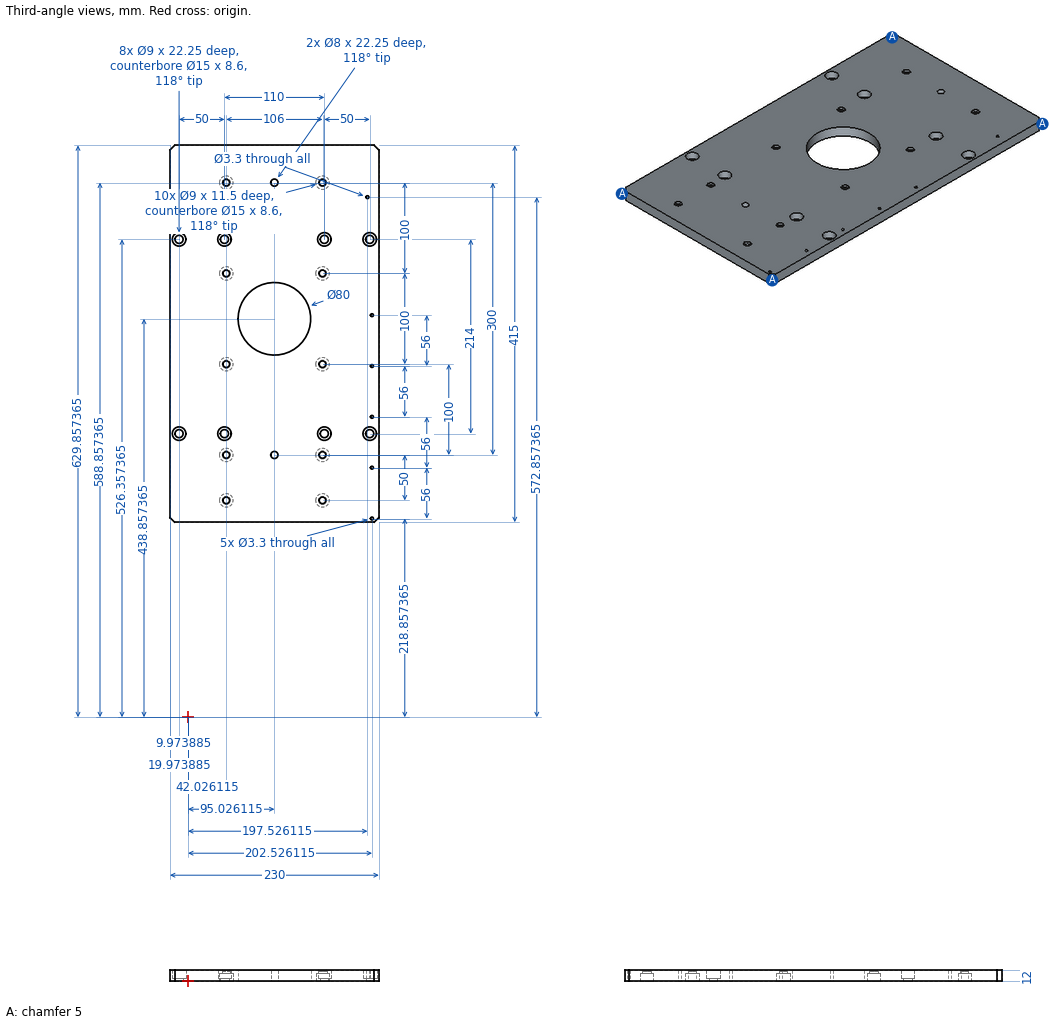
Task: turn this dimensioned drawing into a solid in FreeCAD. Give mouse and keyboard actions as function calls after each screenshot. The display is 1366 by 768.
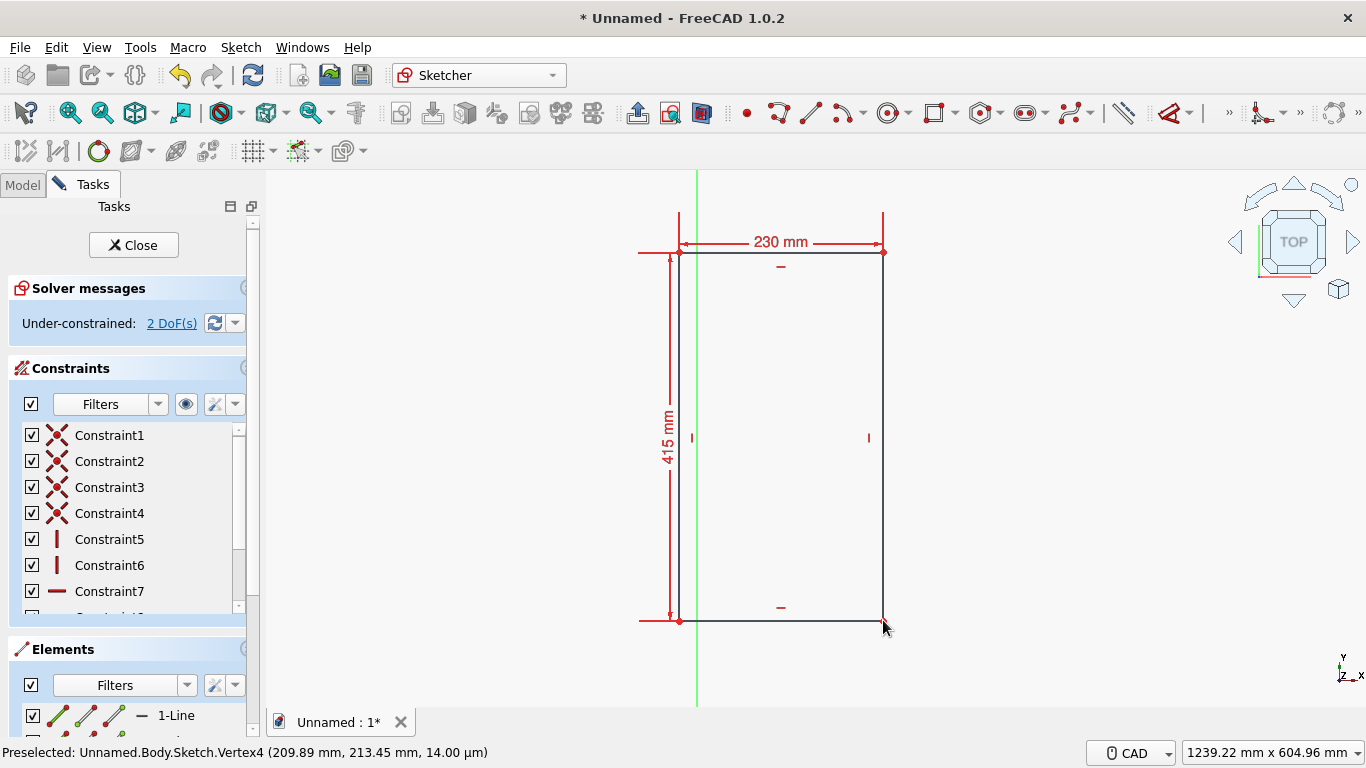
click(1170, 114)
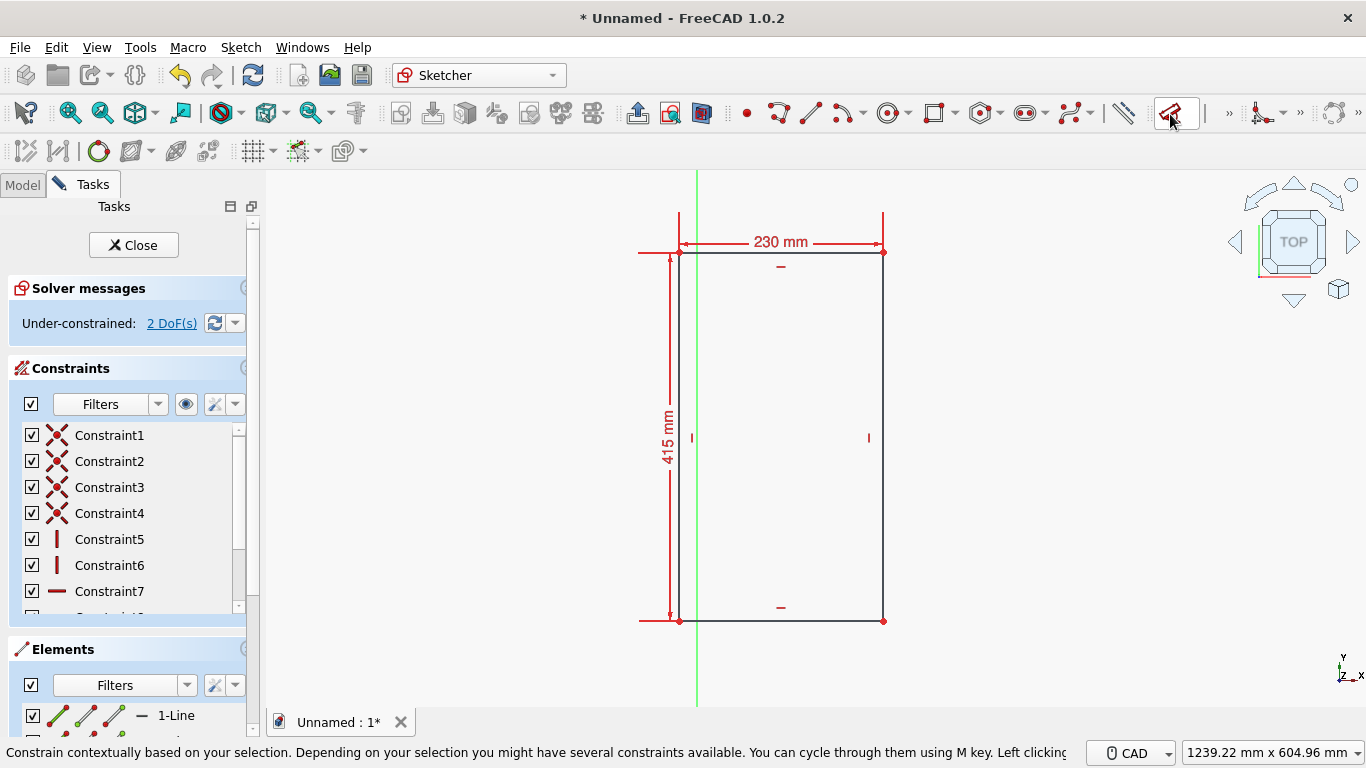
scroll(679, 253, up, 5)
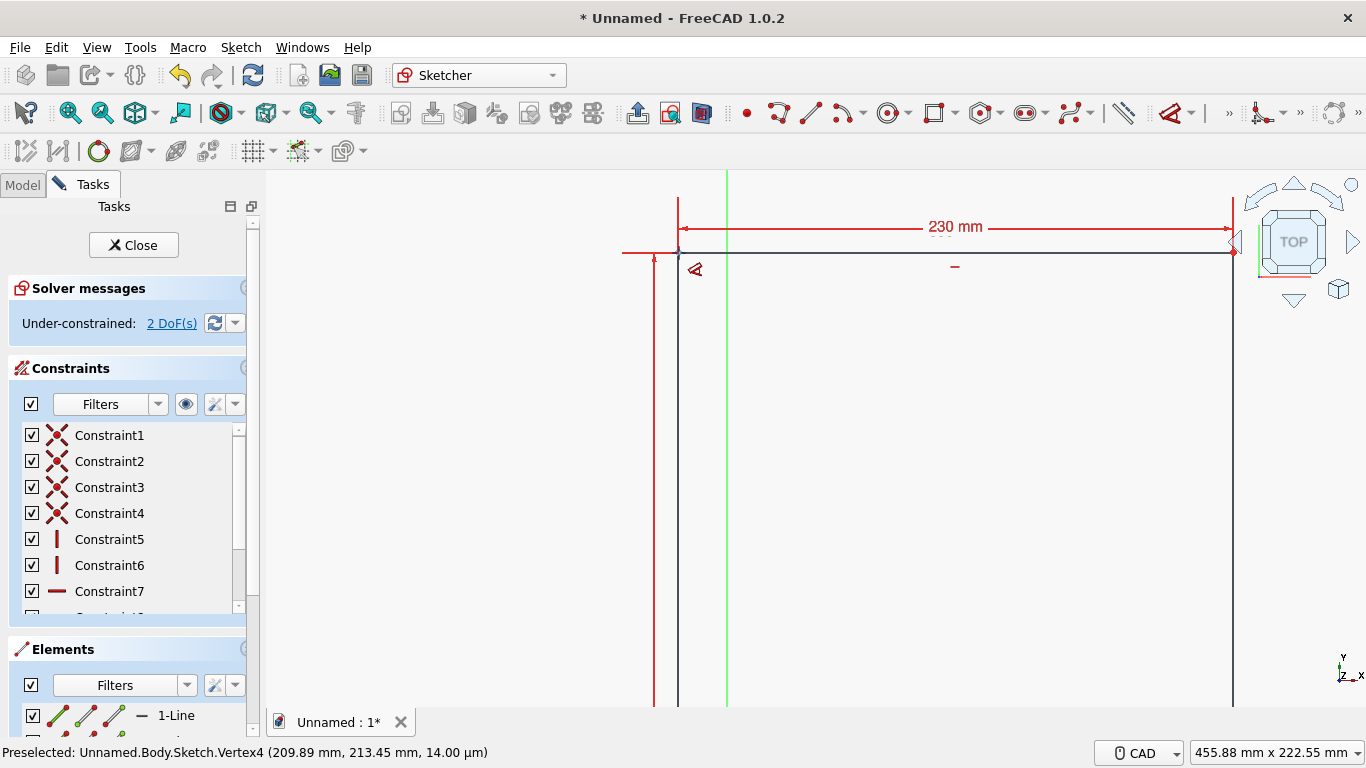
click(678, 253)
click(703, 219)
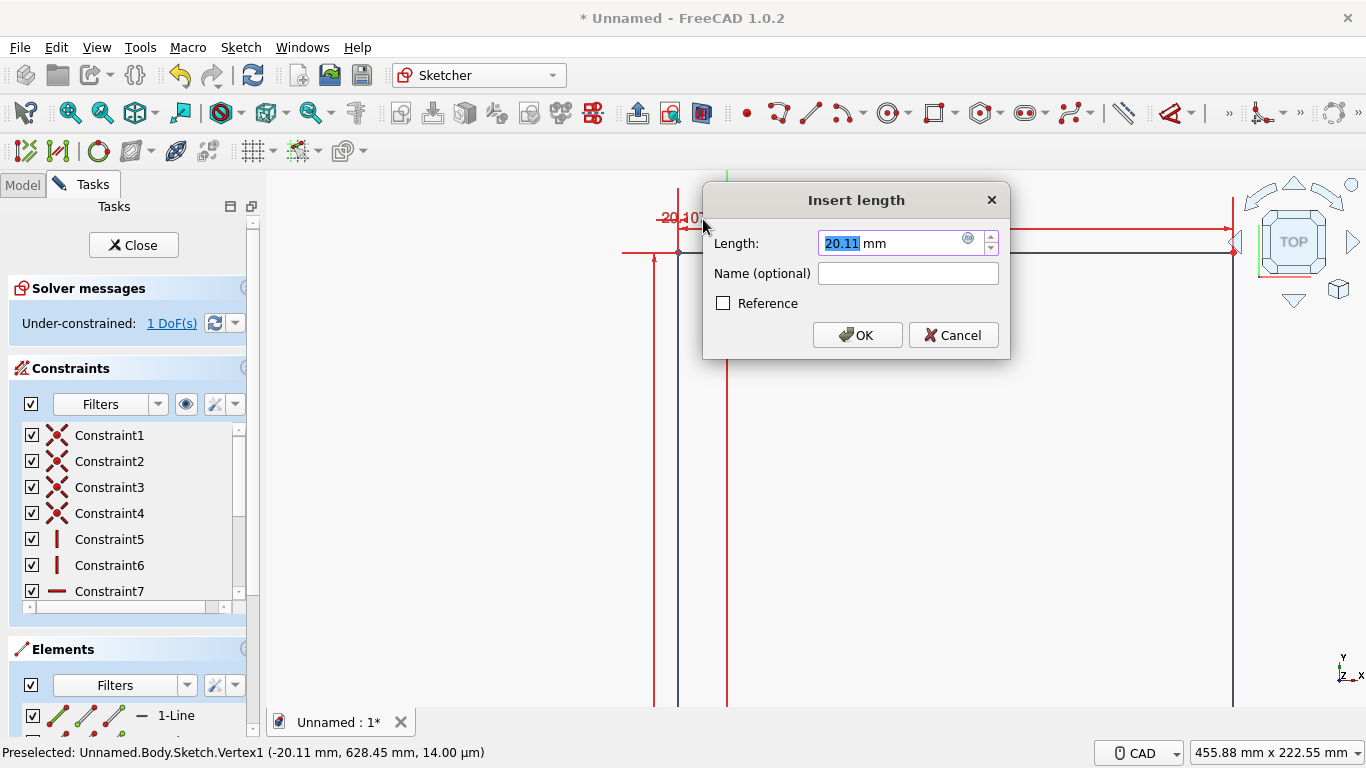
text(19.973885)
key(Return)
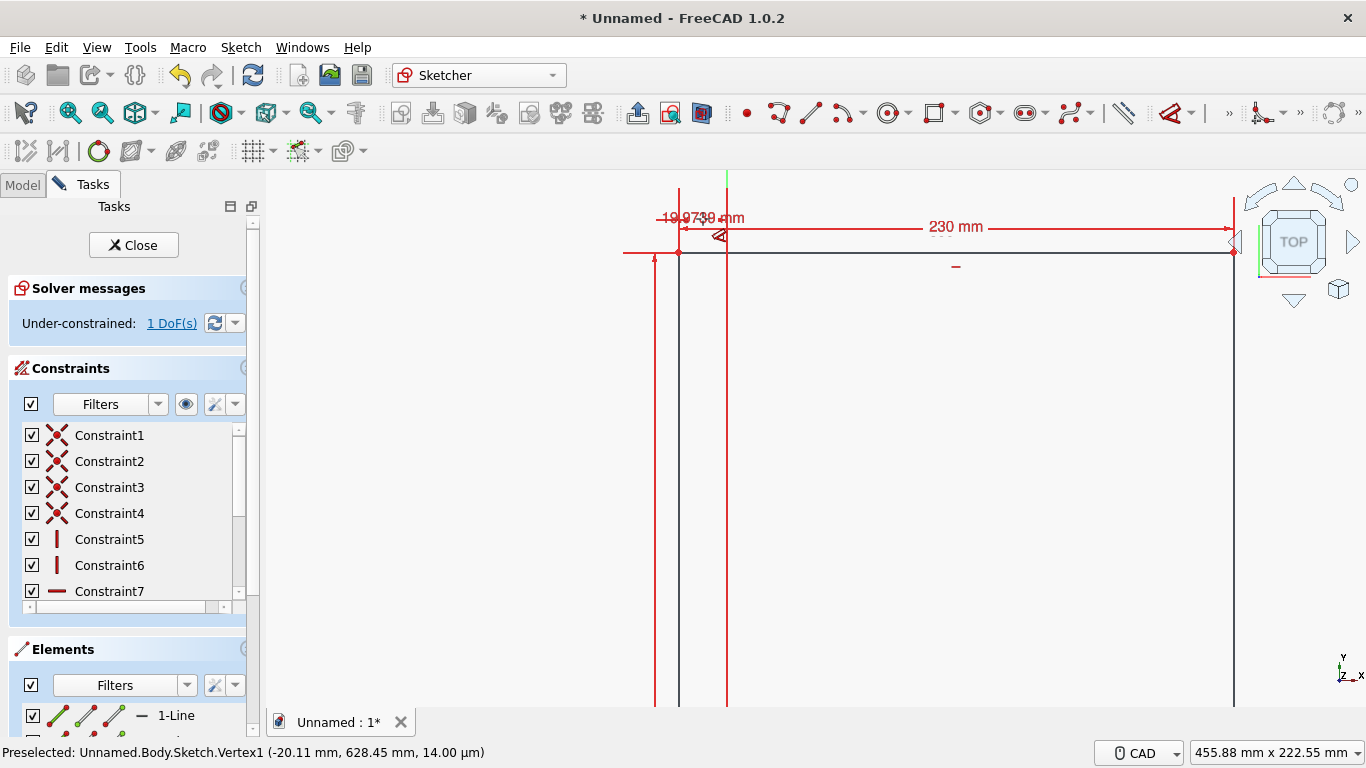
scroll(679, 252, down, 7)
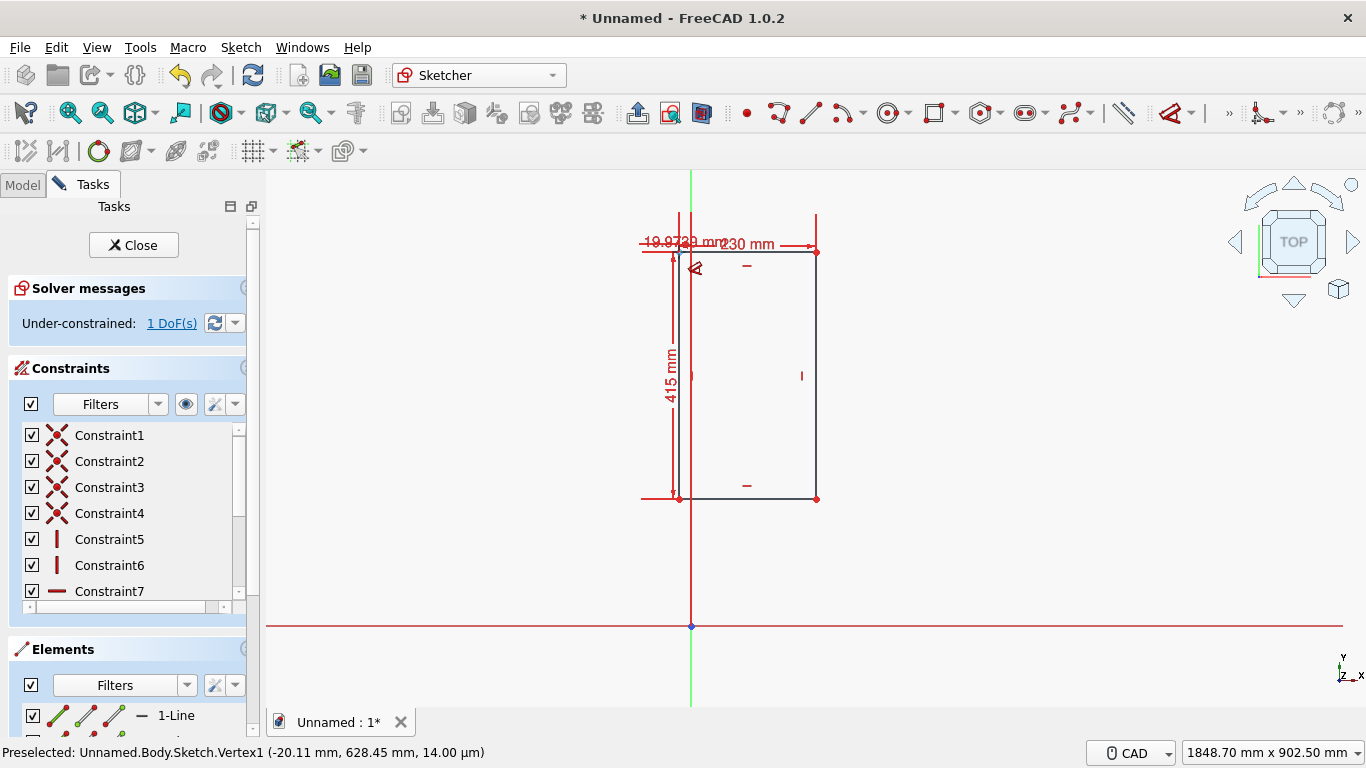
click(679, 252)
click(645, 439)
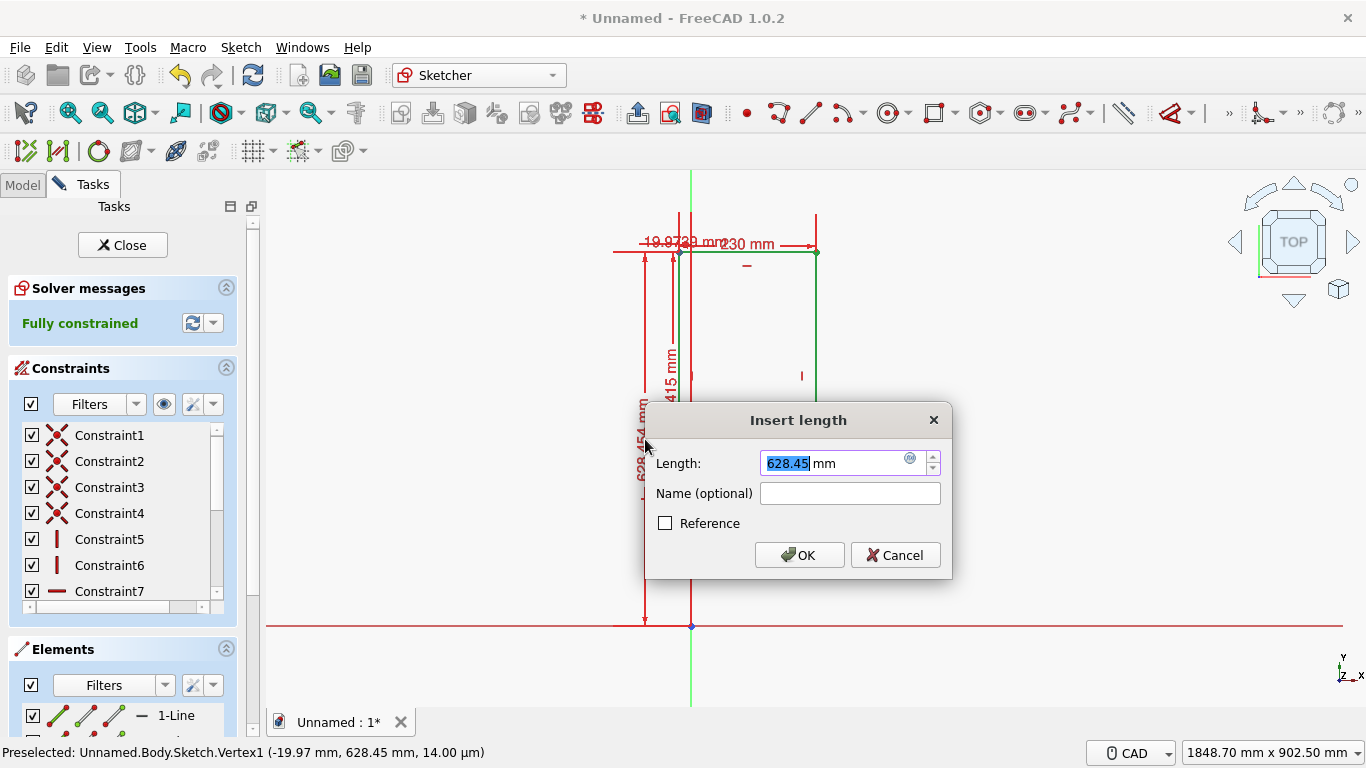
text(629.857365)
key(Return)
key(Escape)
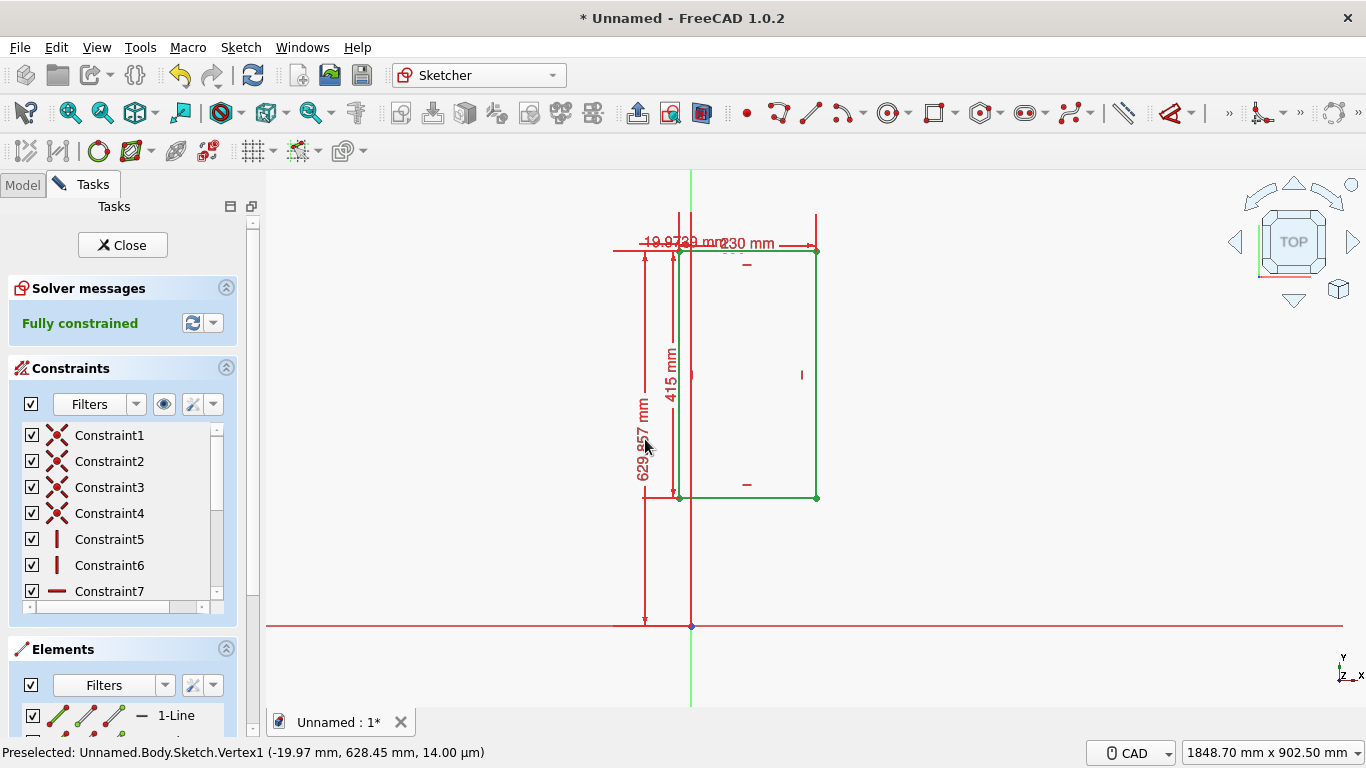
click(123, 245)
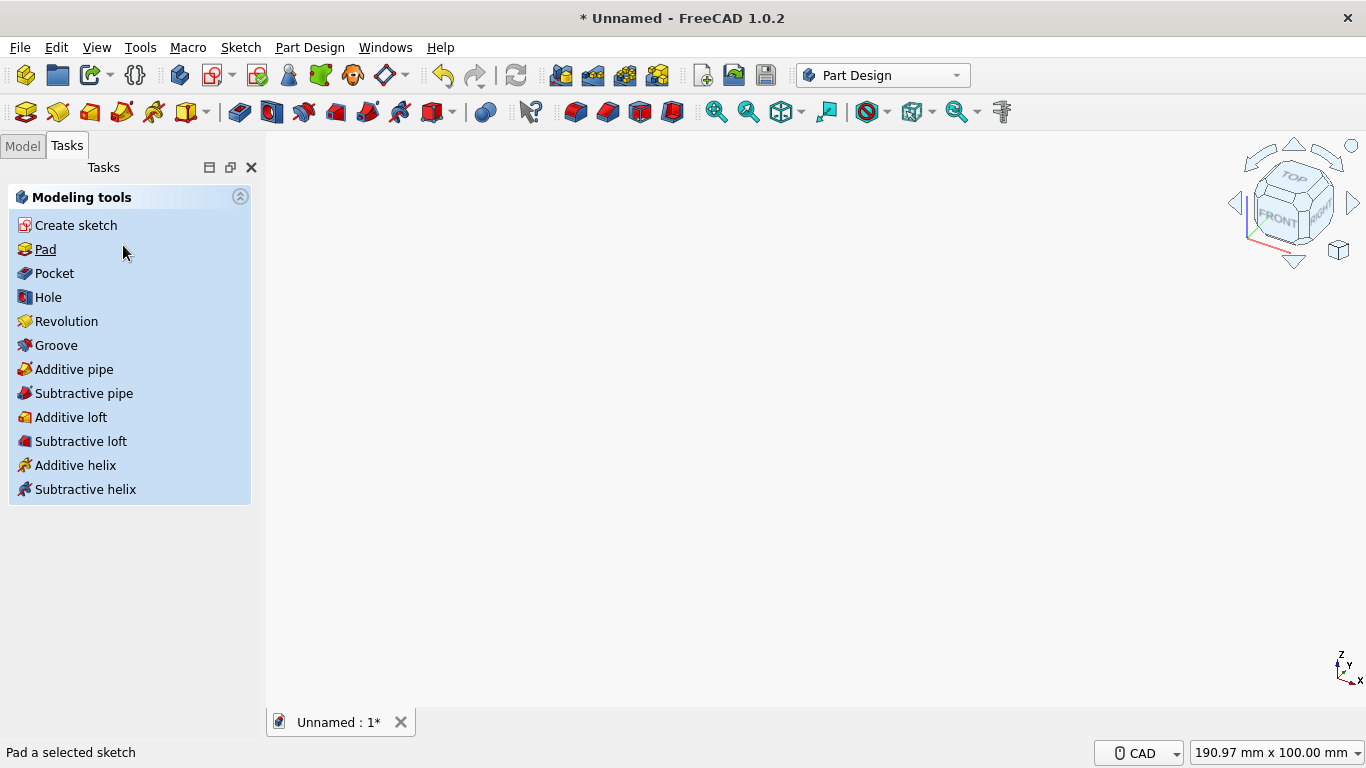
click(26, 112)